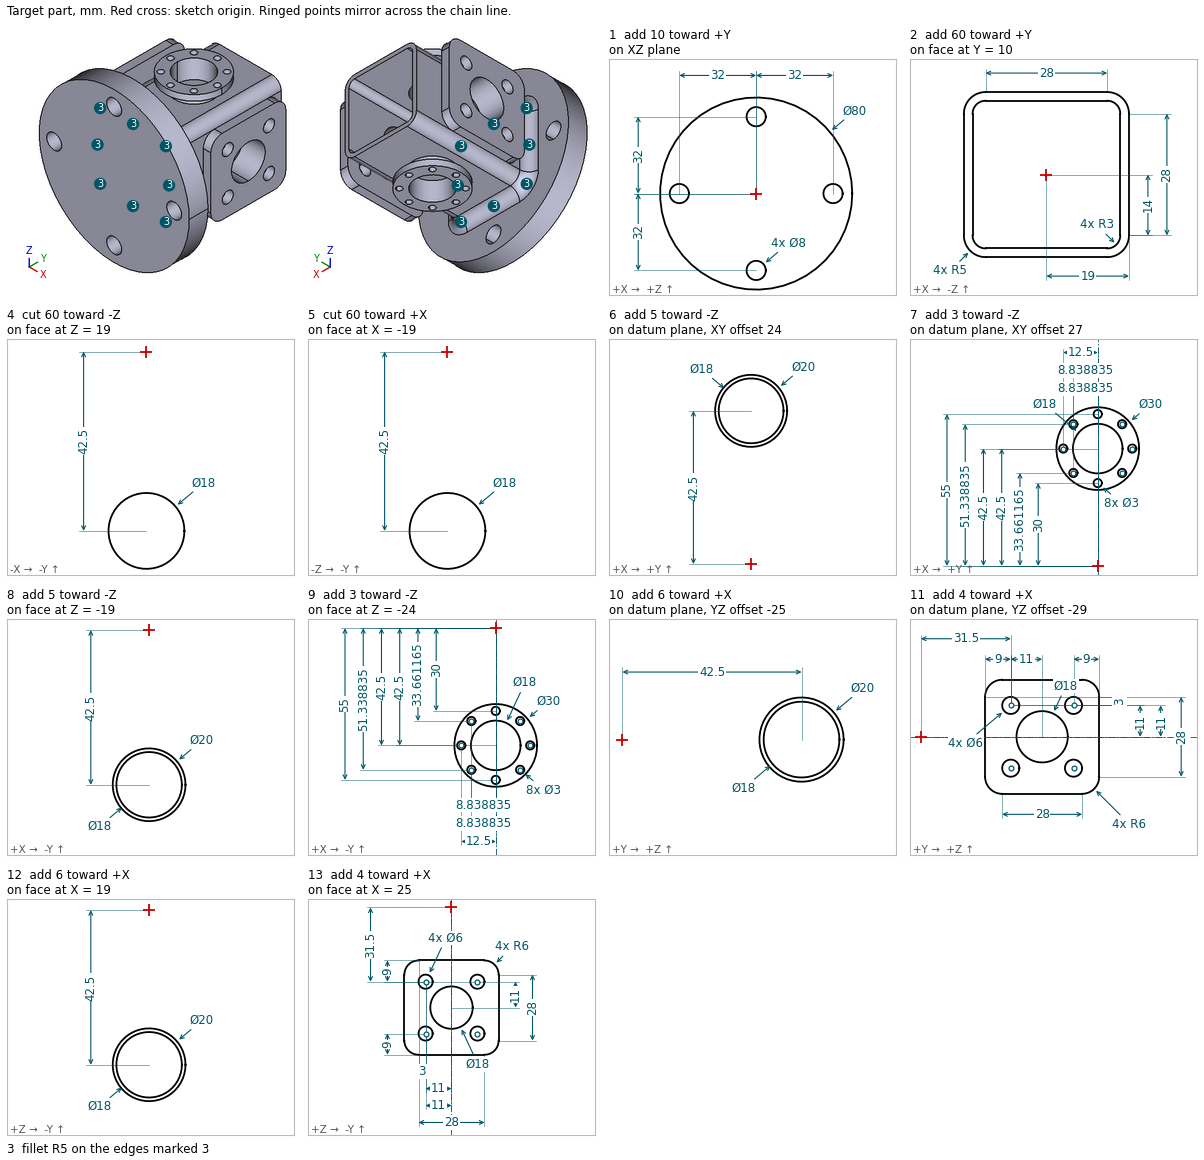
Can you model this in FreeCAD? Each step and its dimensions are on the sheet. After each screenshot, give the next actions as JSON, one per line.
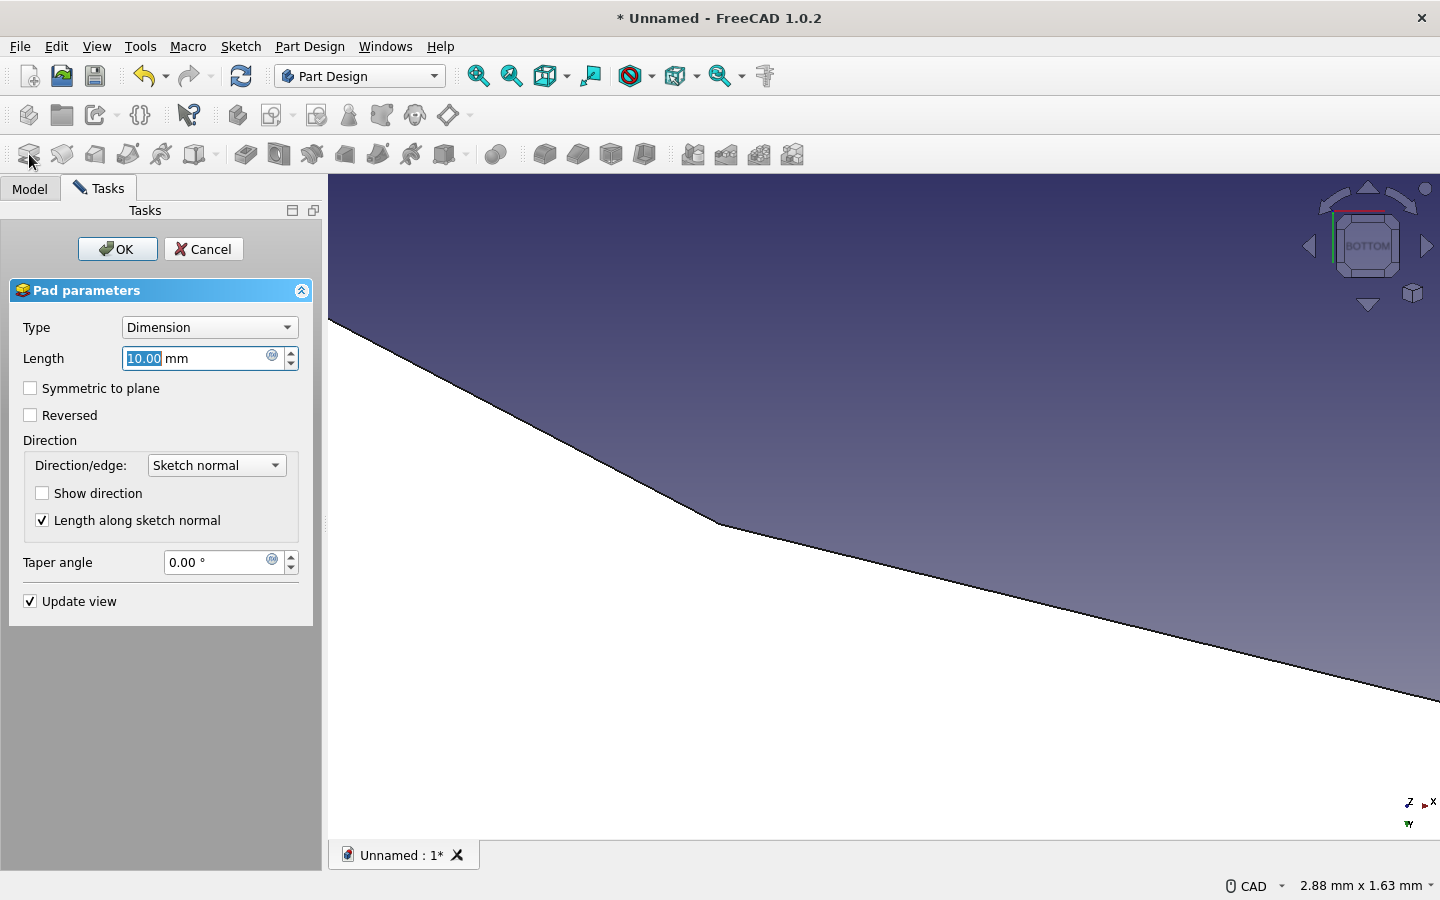
{"action": "type", "text": "3"}
{"action": "key", "text": "Tab"}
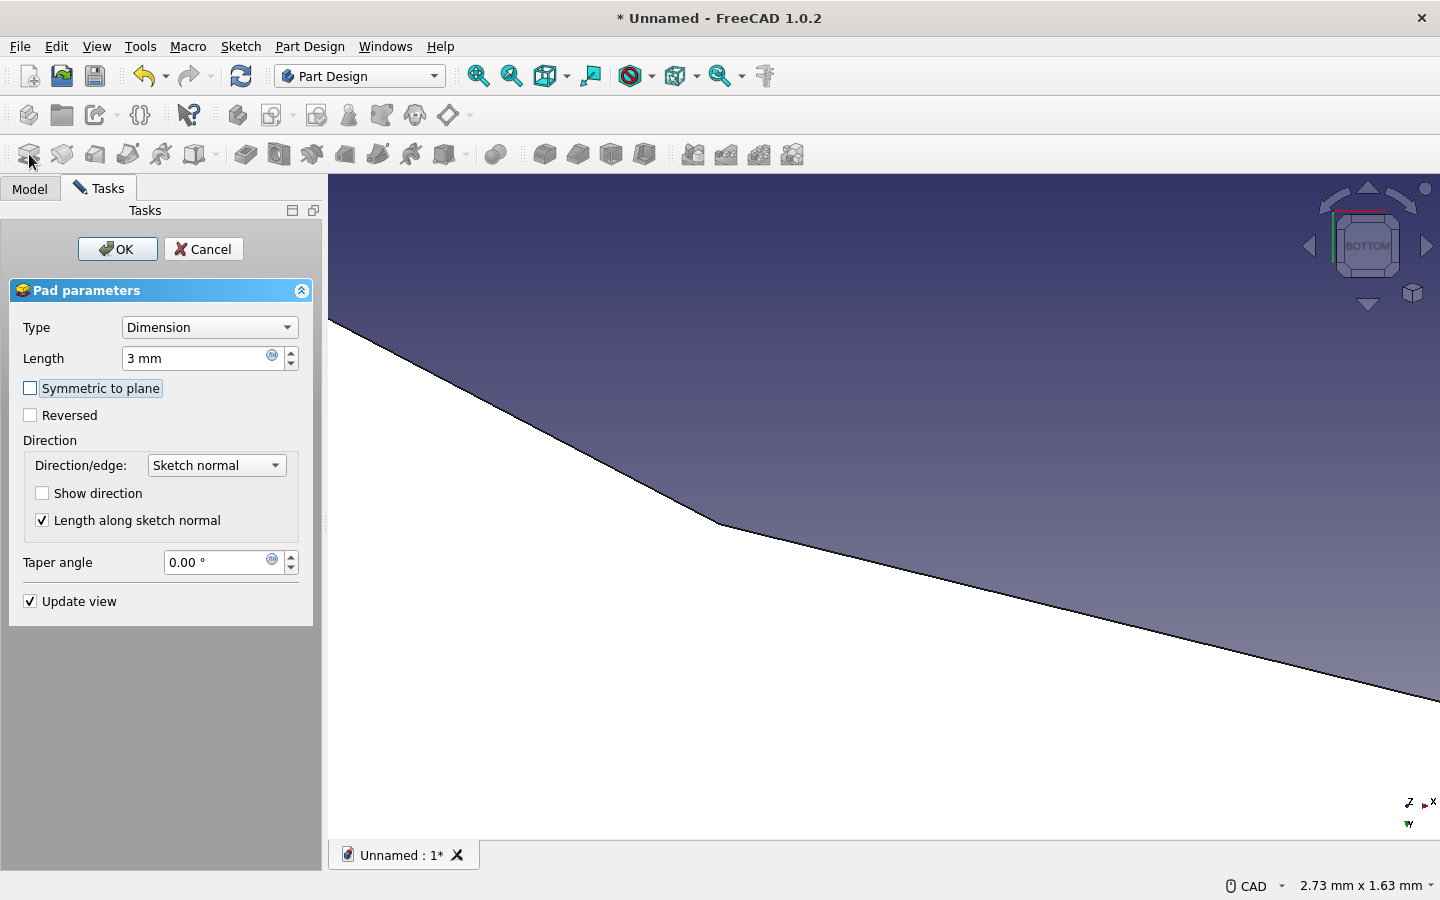
{"action": "left_click", "coordinate": [118, 249]}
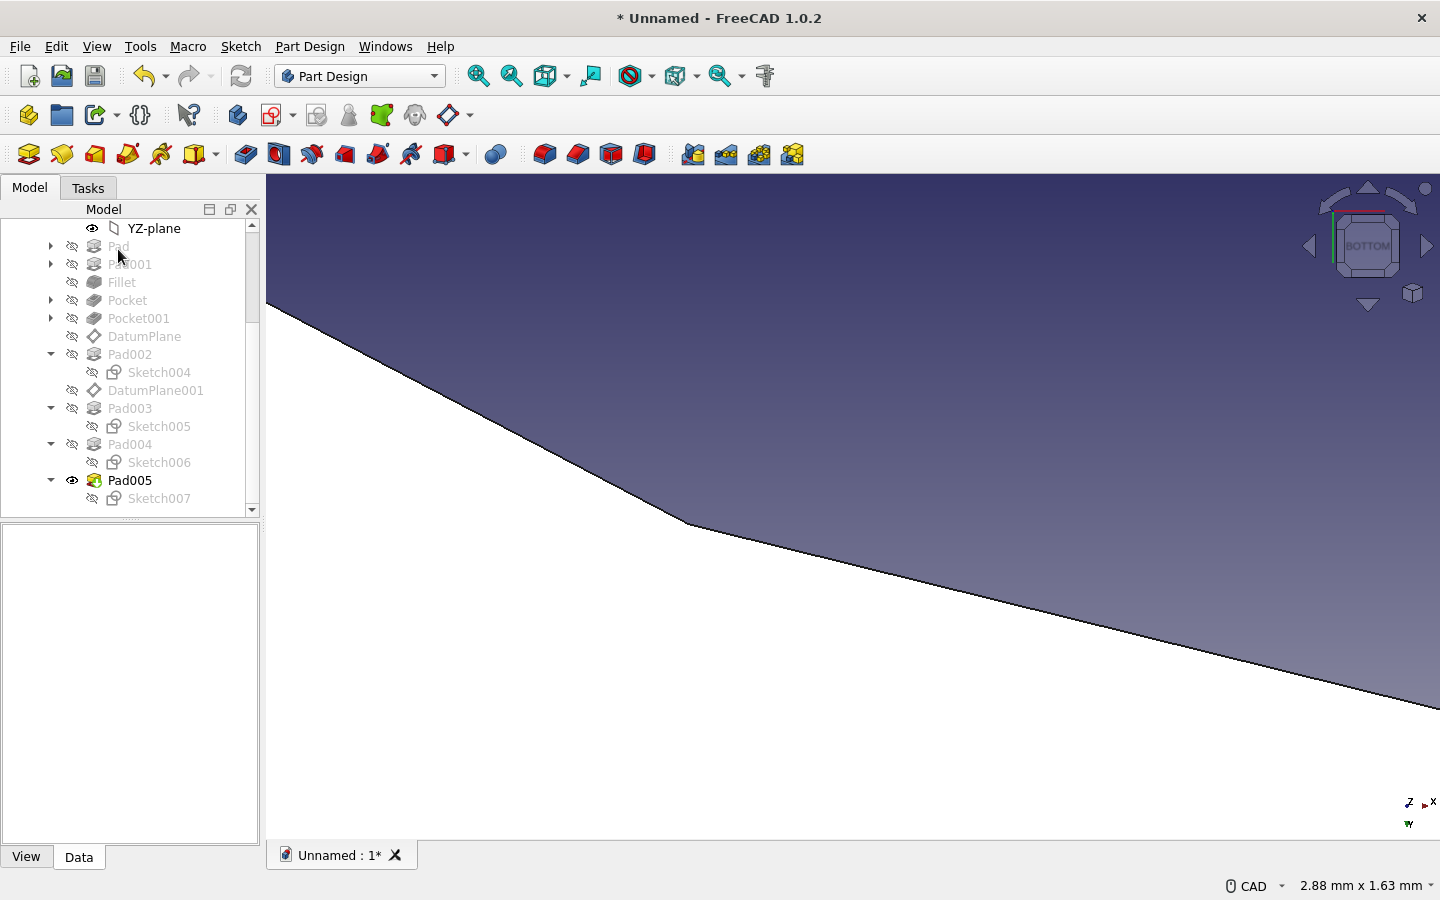
{"action": "key", "text": "v f"}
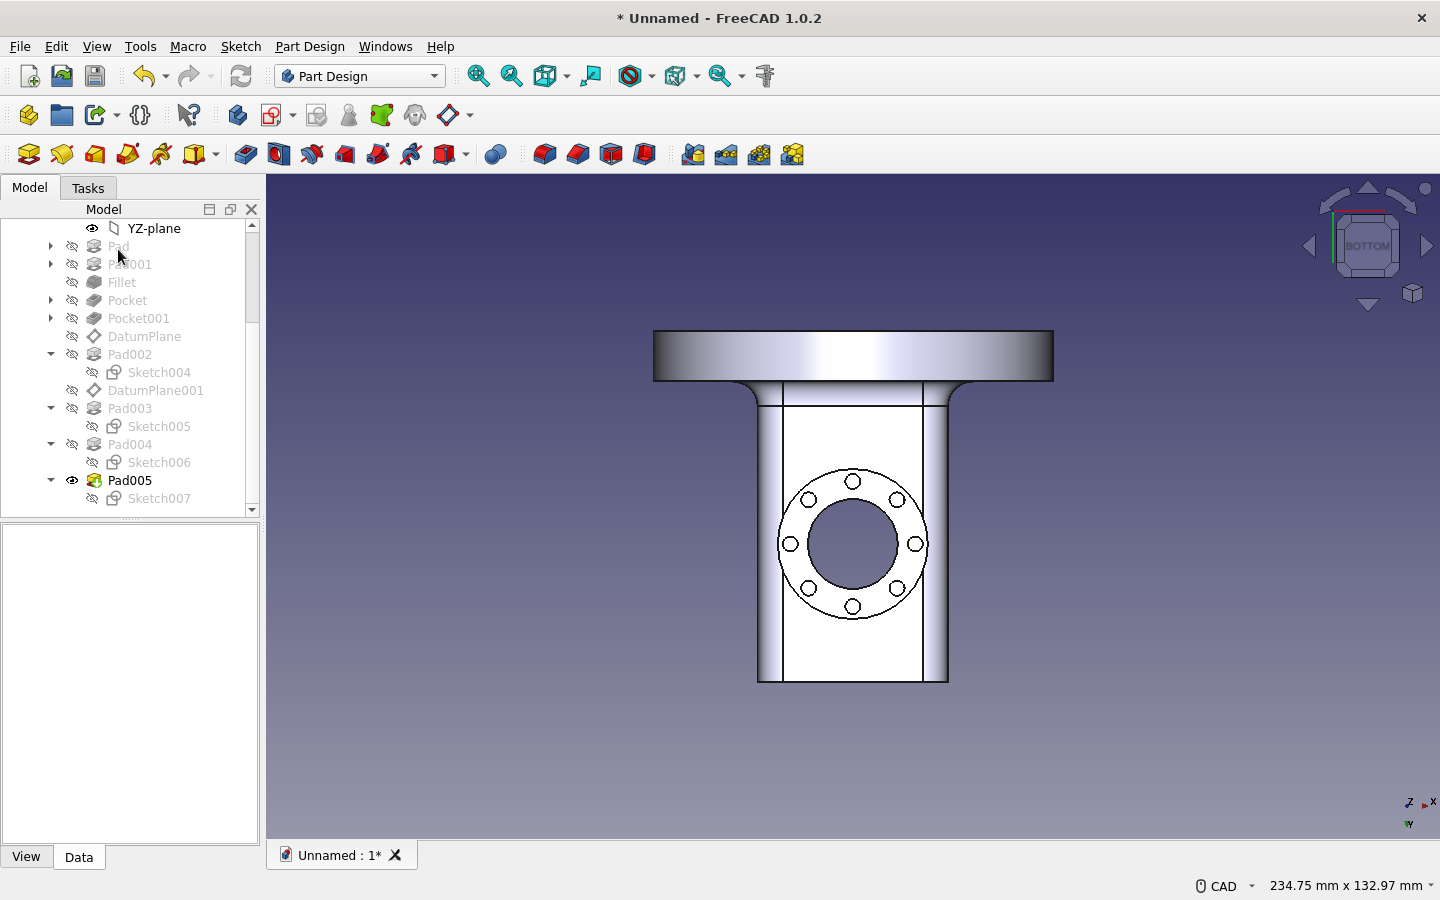
{"action": "scroll", "coordinate": [161, 368], "scroll_direction": "down", "scroll_amount": 3}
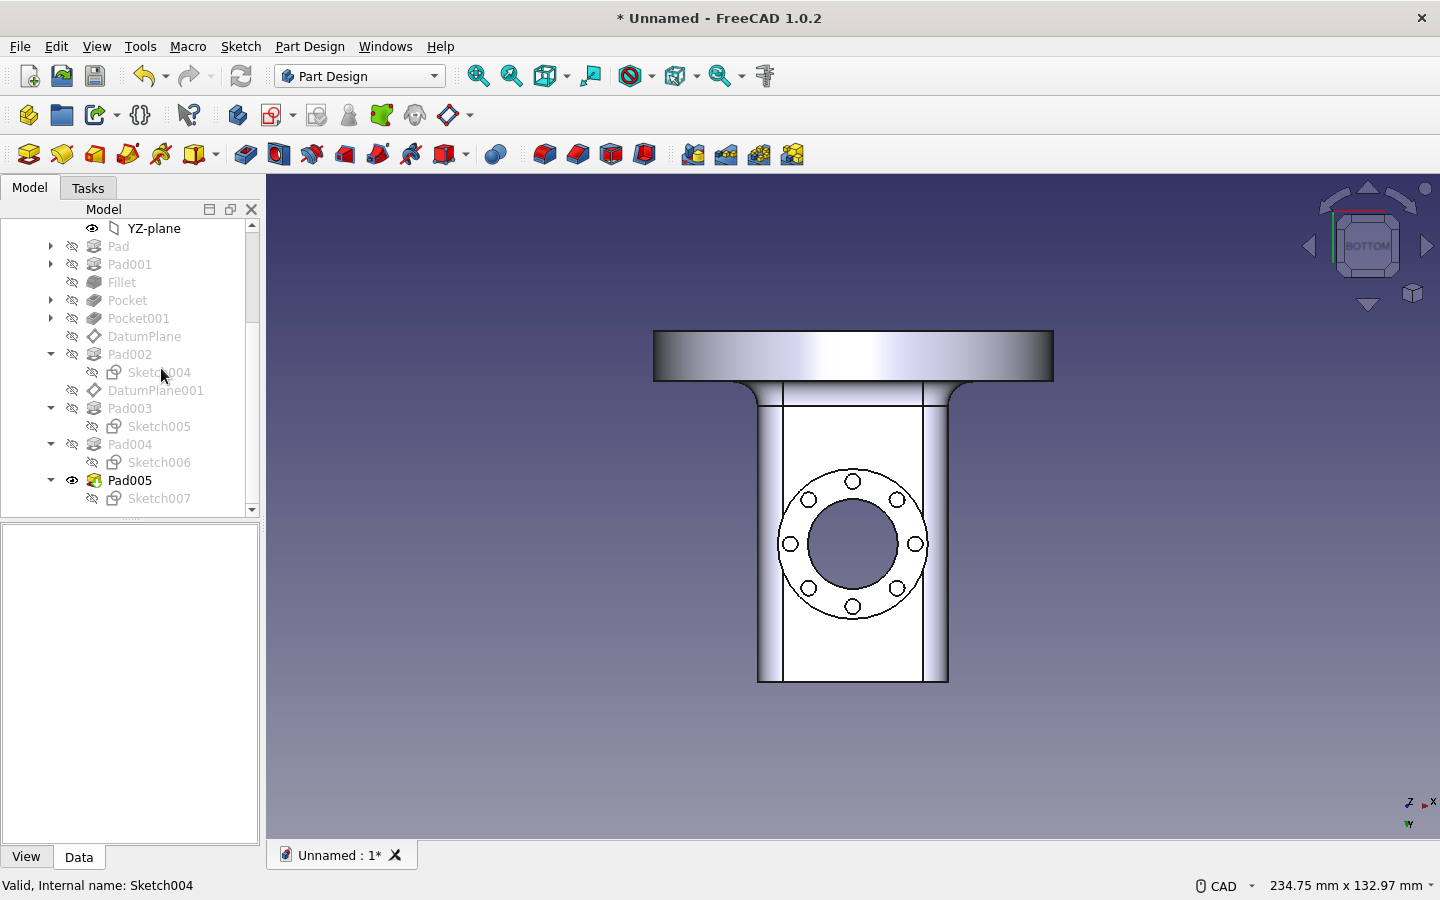
{"action": "scroll", "coordinate": [161, 368], "scroll_direction": "up", "scroll_amount": 15}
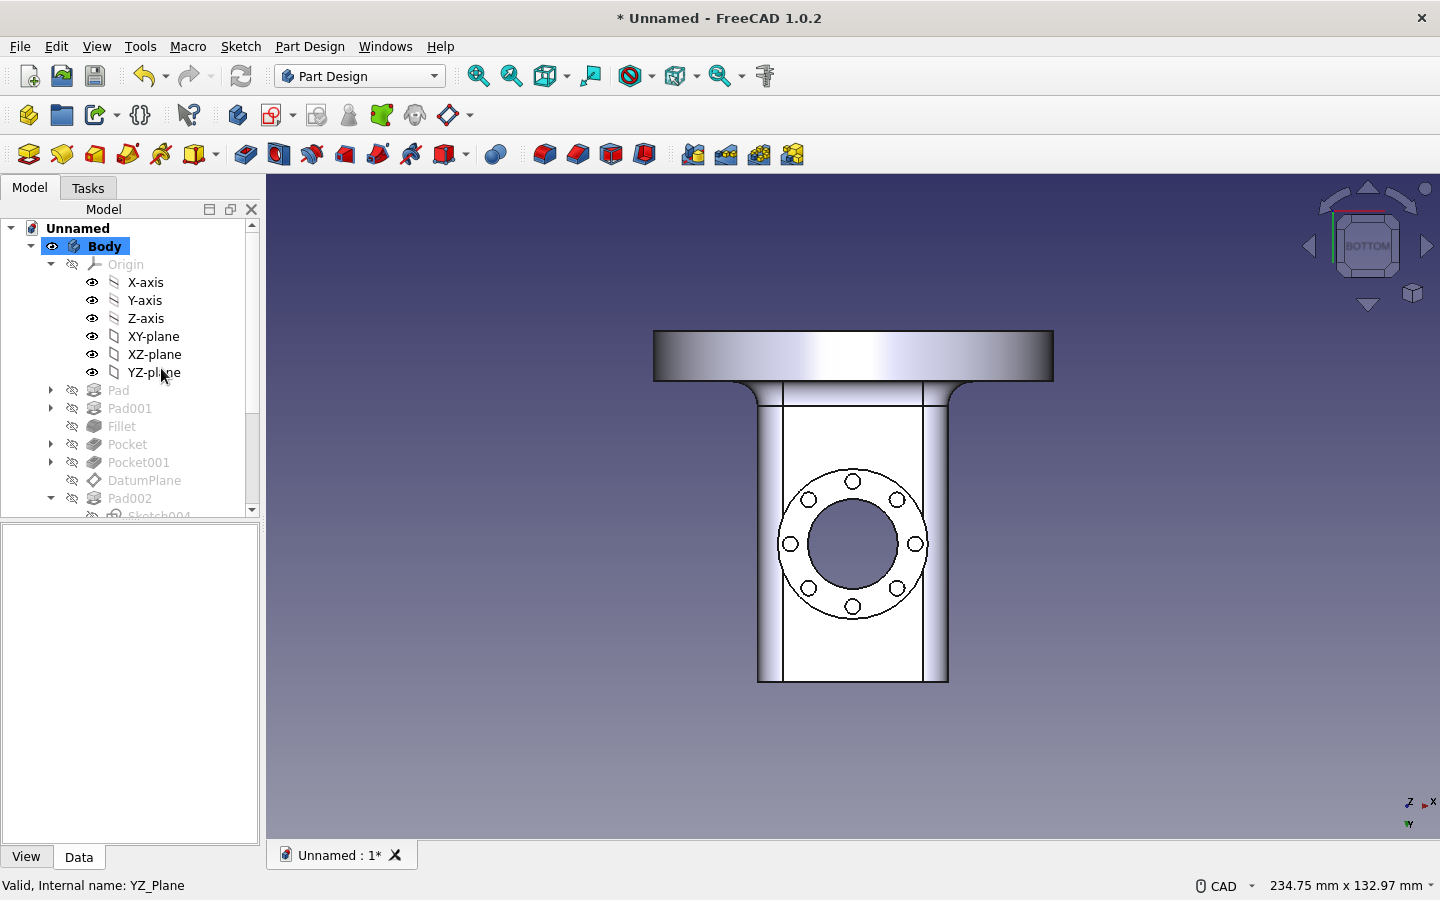
{"action": "left_click", "coordinate": [137, 372]}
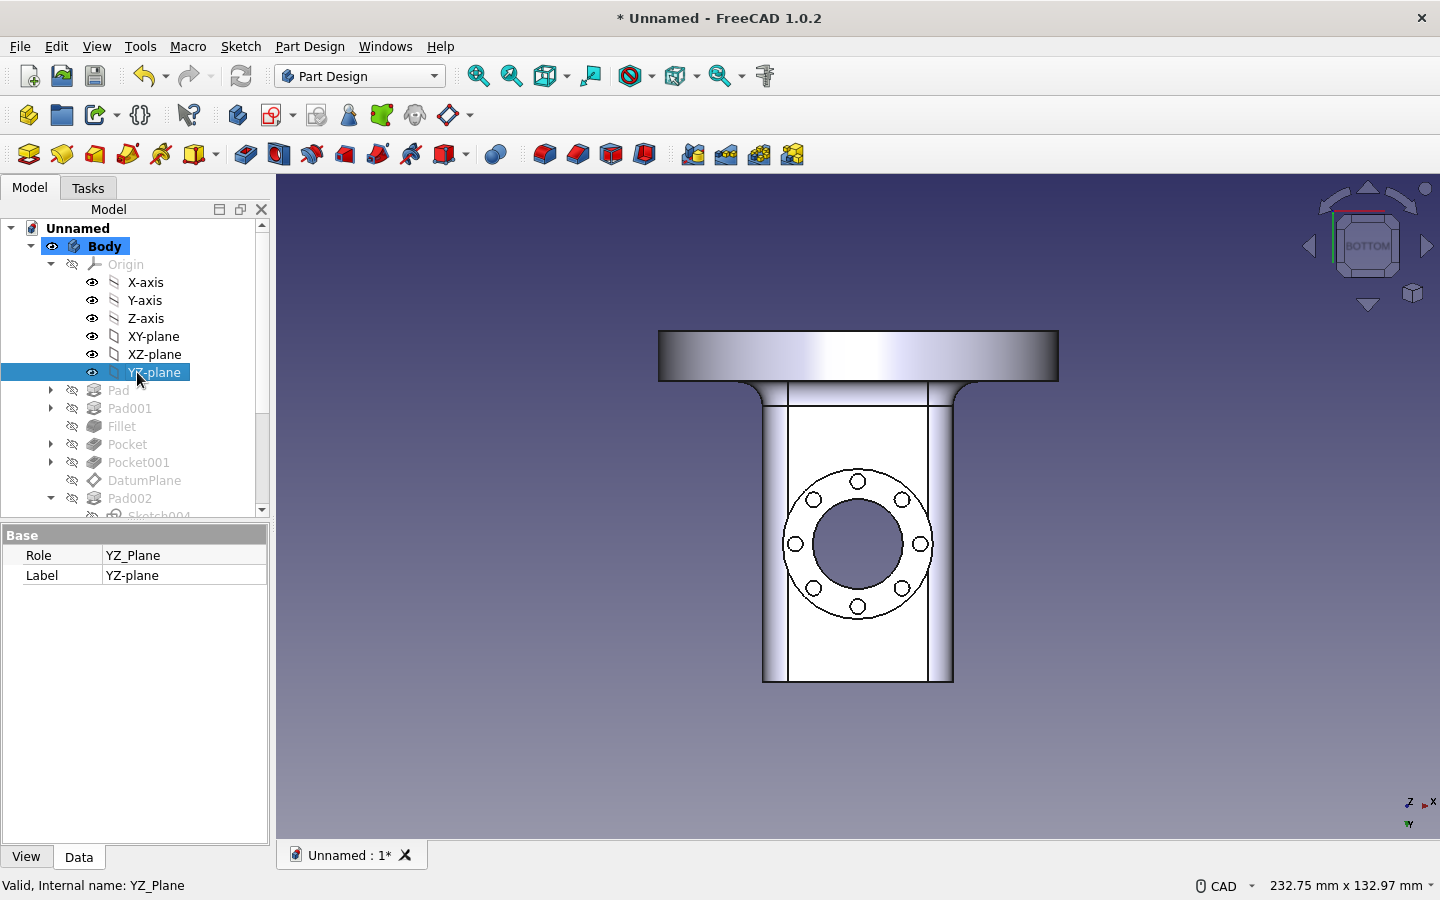
{"action": "left_click", "coordinate": [448, 116]}